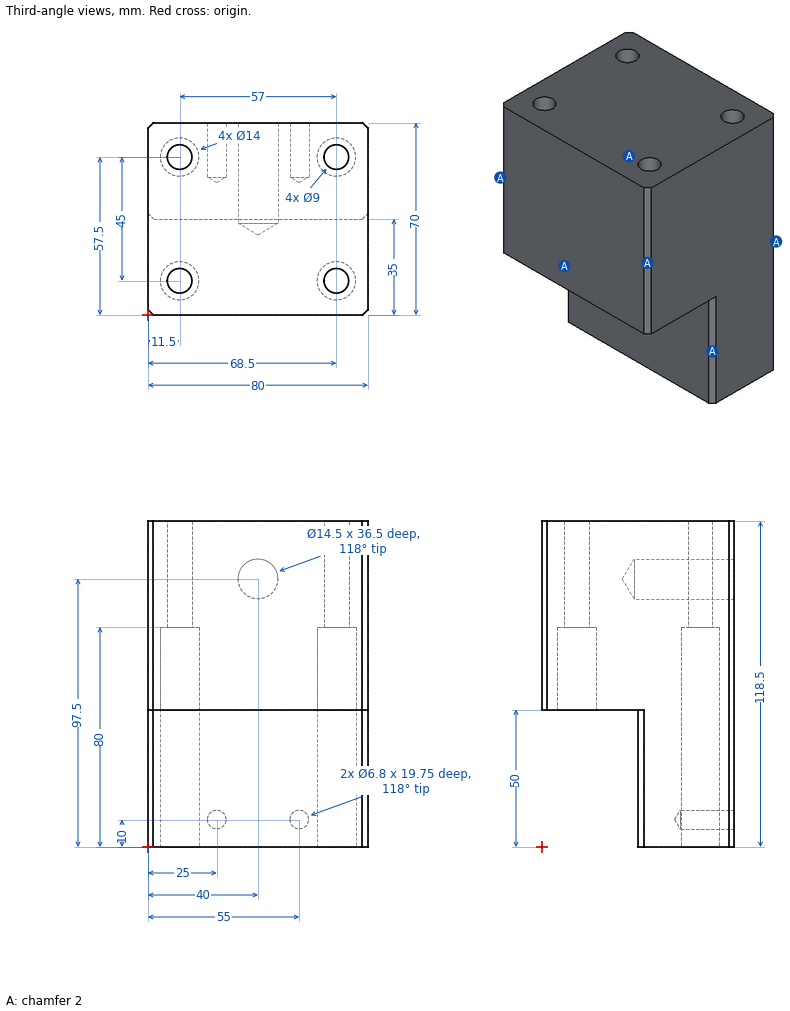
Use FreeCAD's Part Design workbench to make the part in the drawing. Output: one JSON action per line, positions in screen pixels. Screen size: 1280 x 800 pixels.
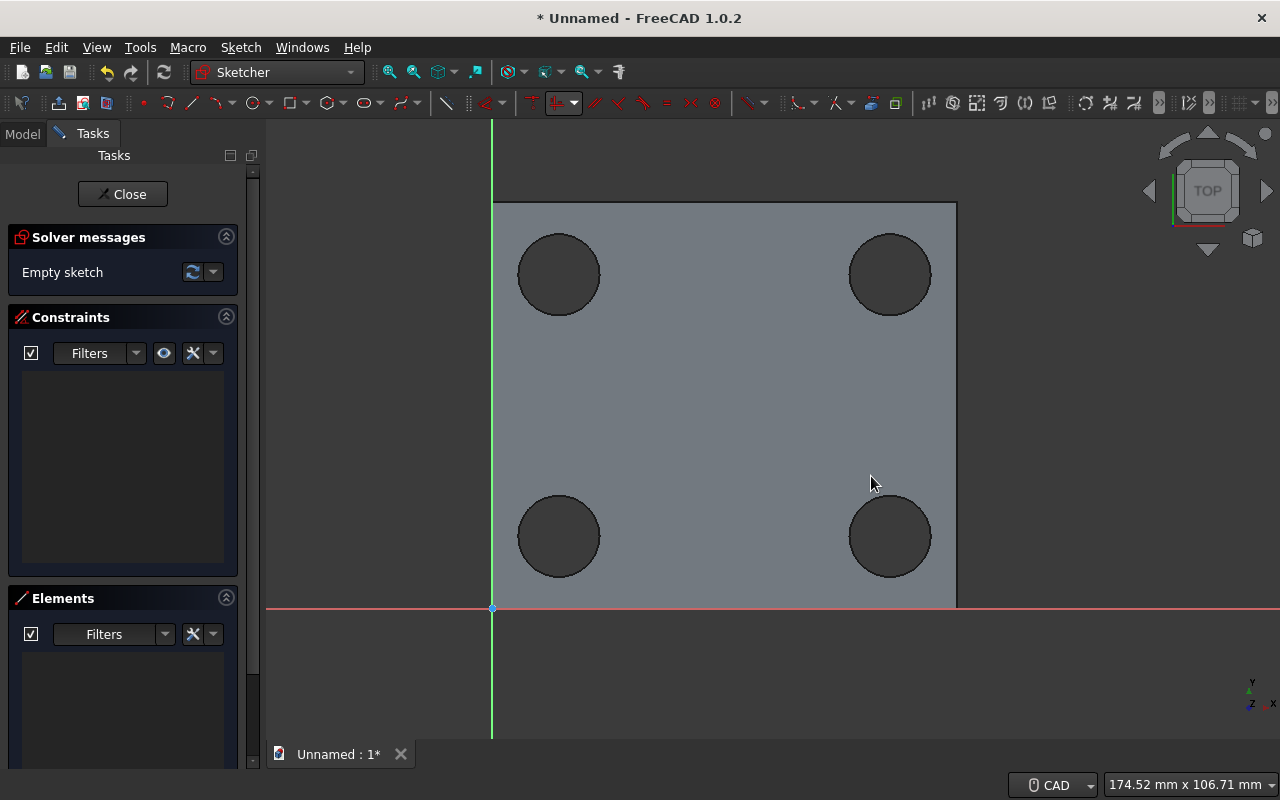
{"action": "left_click", "coordinate": [254, 104]}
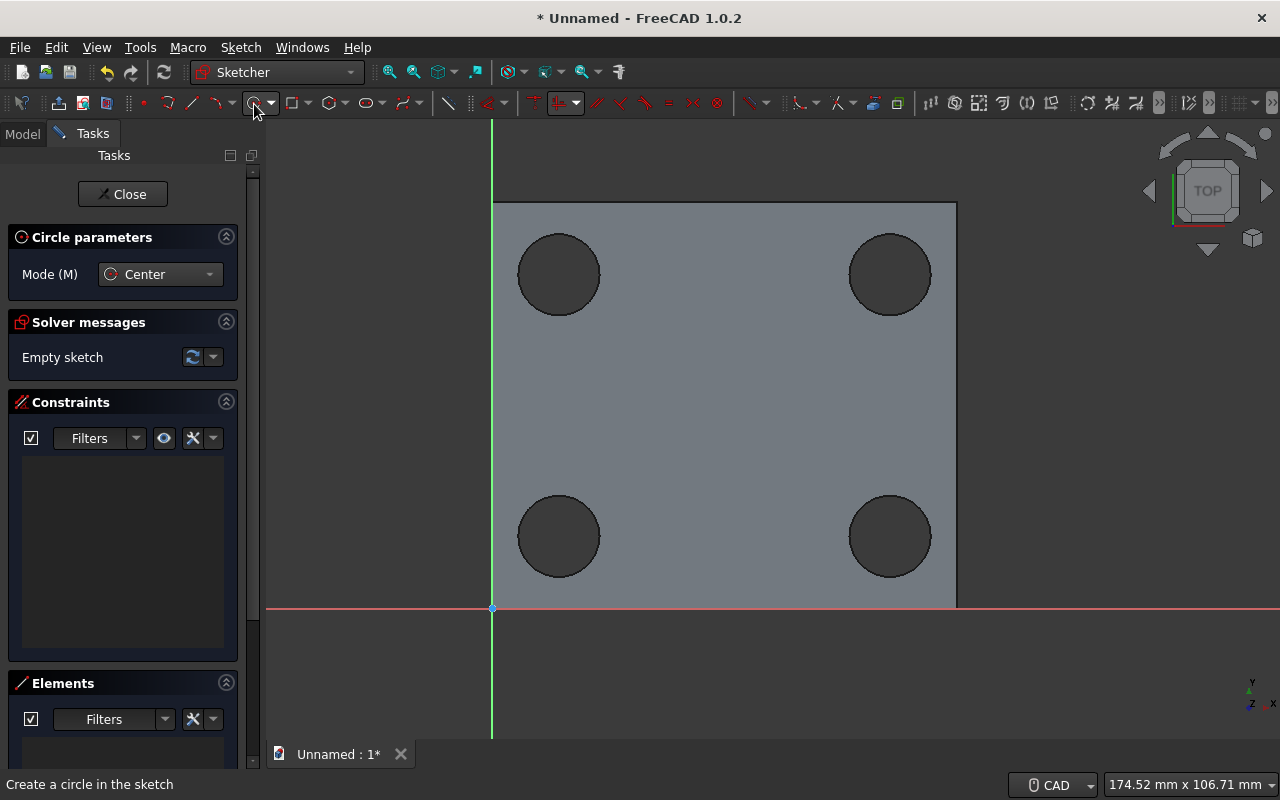
{"action": "left_click", "coordinate": [890, 275]}
{"action": "left_click", "coordinate": [909, 256]}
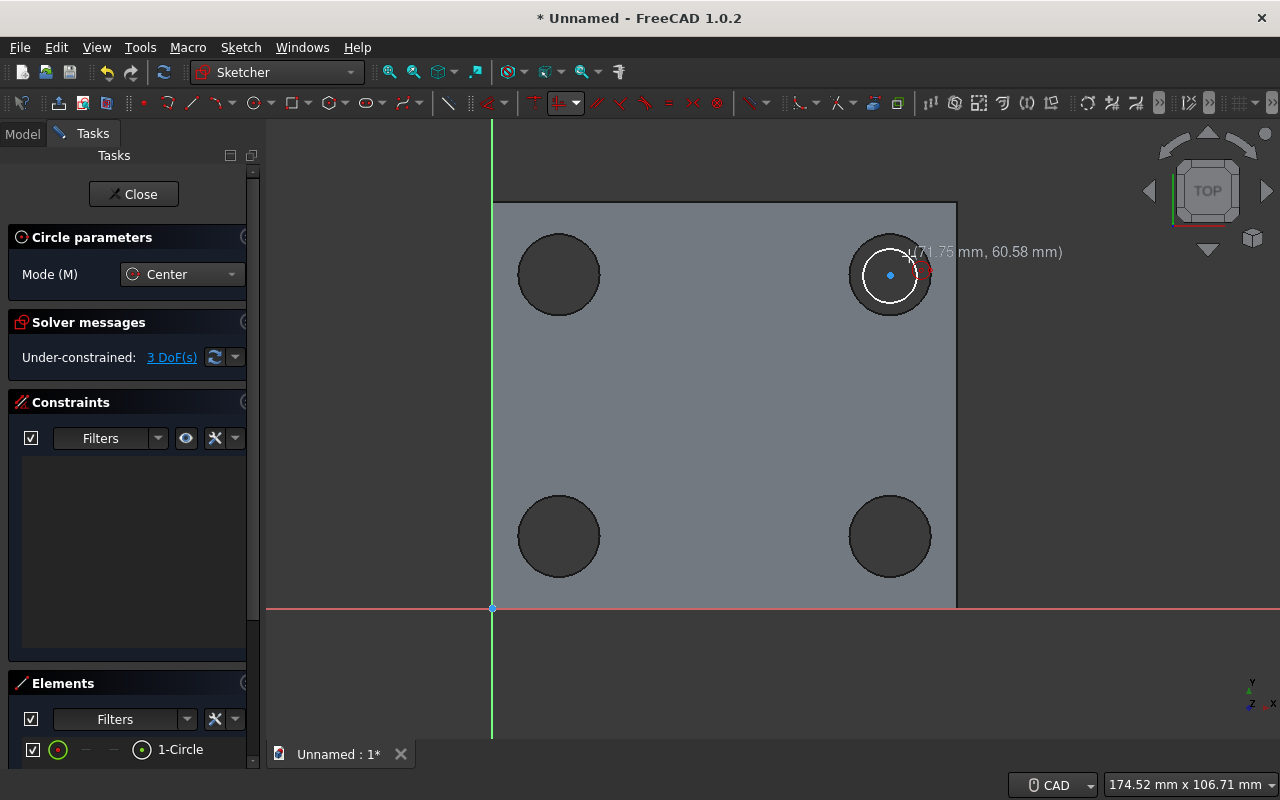
{"action": "left_click", "coordinate": [559, 275]}
{"action": "left_click", "coordinate": [577, 256]}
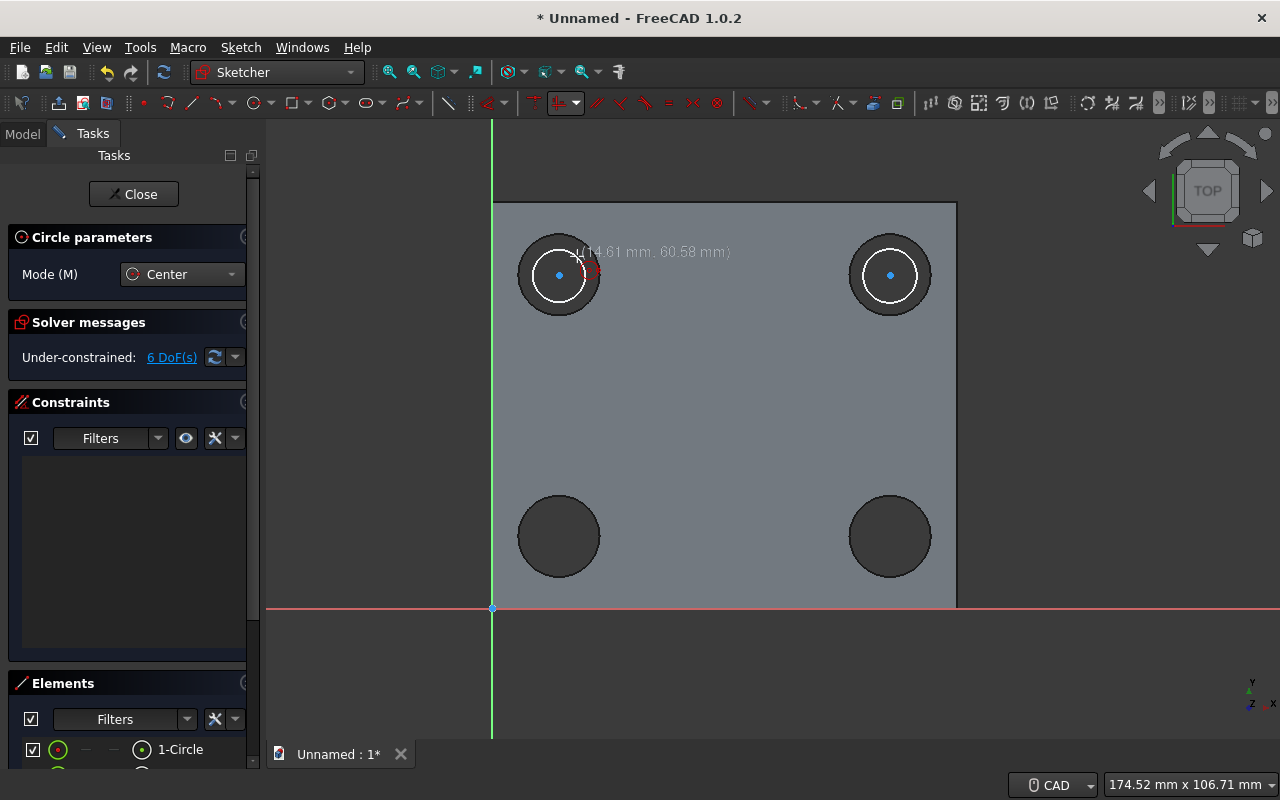
{"action": "left_click", "coordinate": [559, 536]}
{"action": "left_click", "coordinate": [577, 518]}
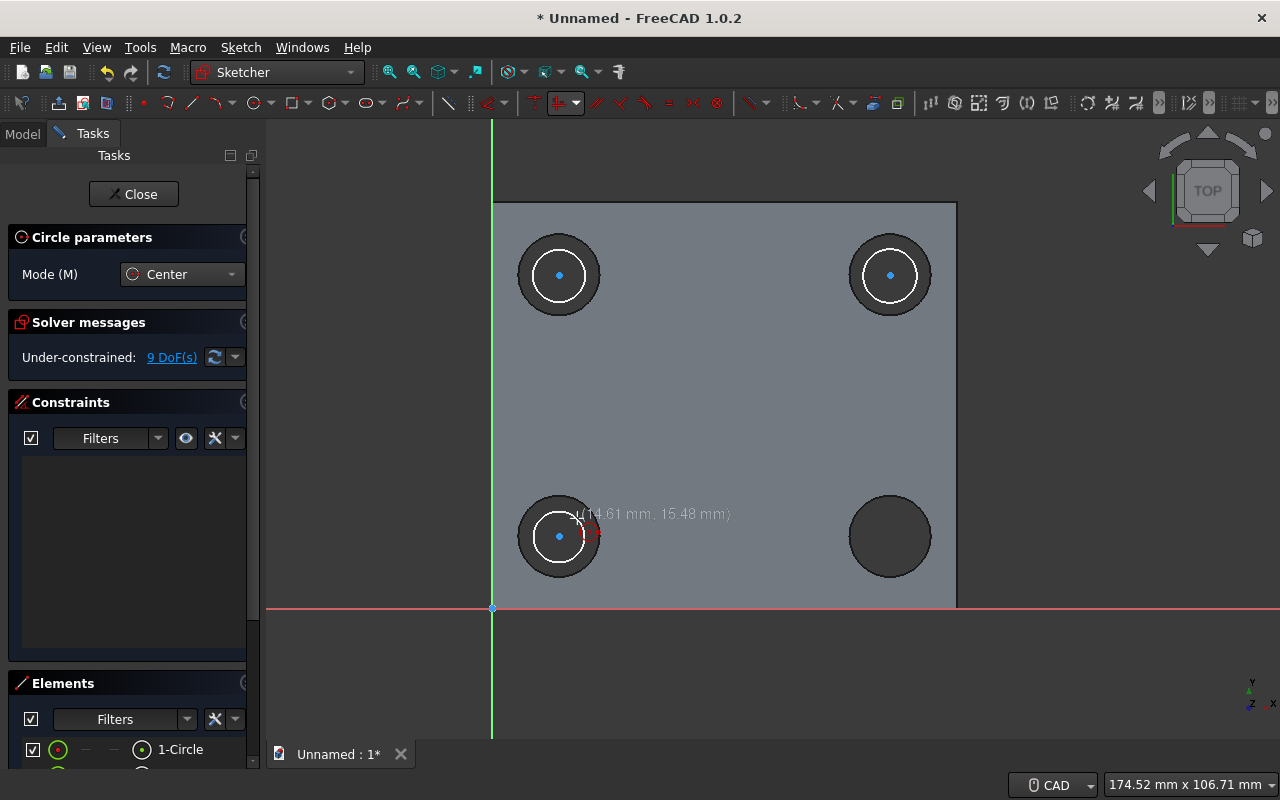
{"action": "left_click", "coordinate": [890, 536]}
{"action": "left_click", "coordinate": [909, 518]}
{"action": "key", "text": "Escape"}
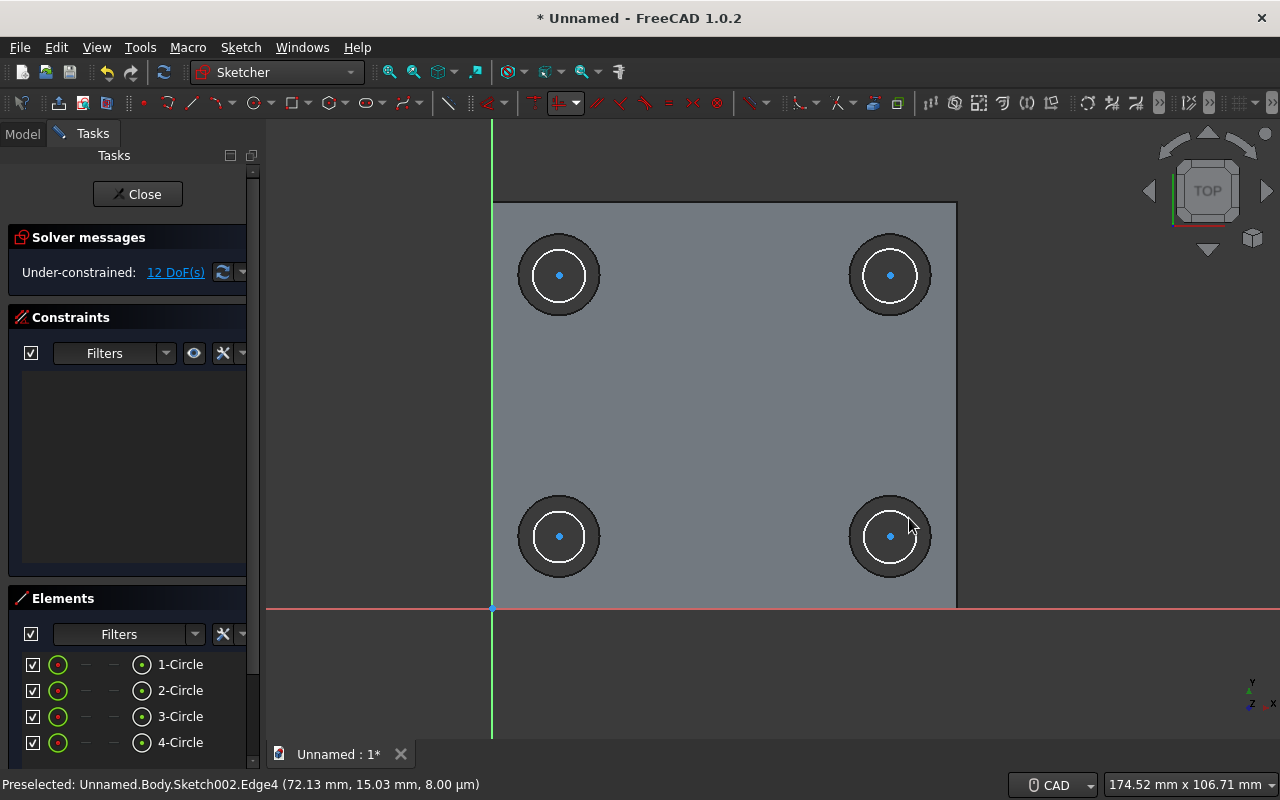
{"action": "left_click", "coordinate": [909, 257]}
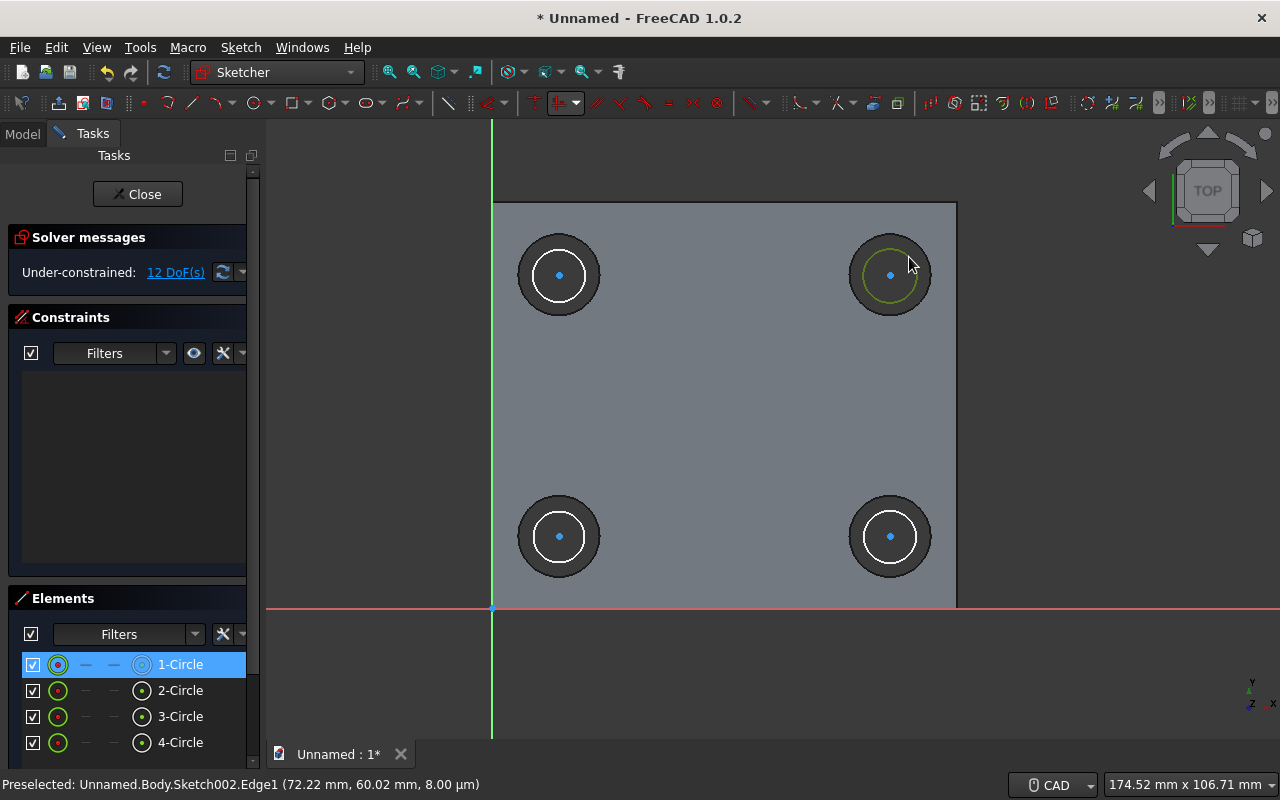
{"action": "left_click", "coordinate": [577, 257]}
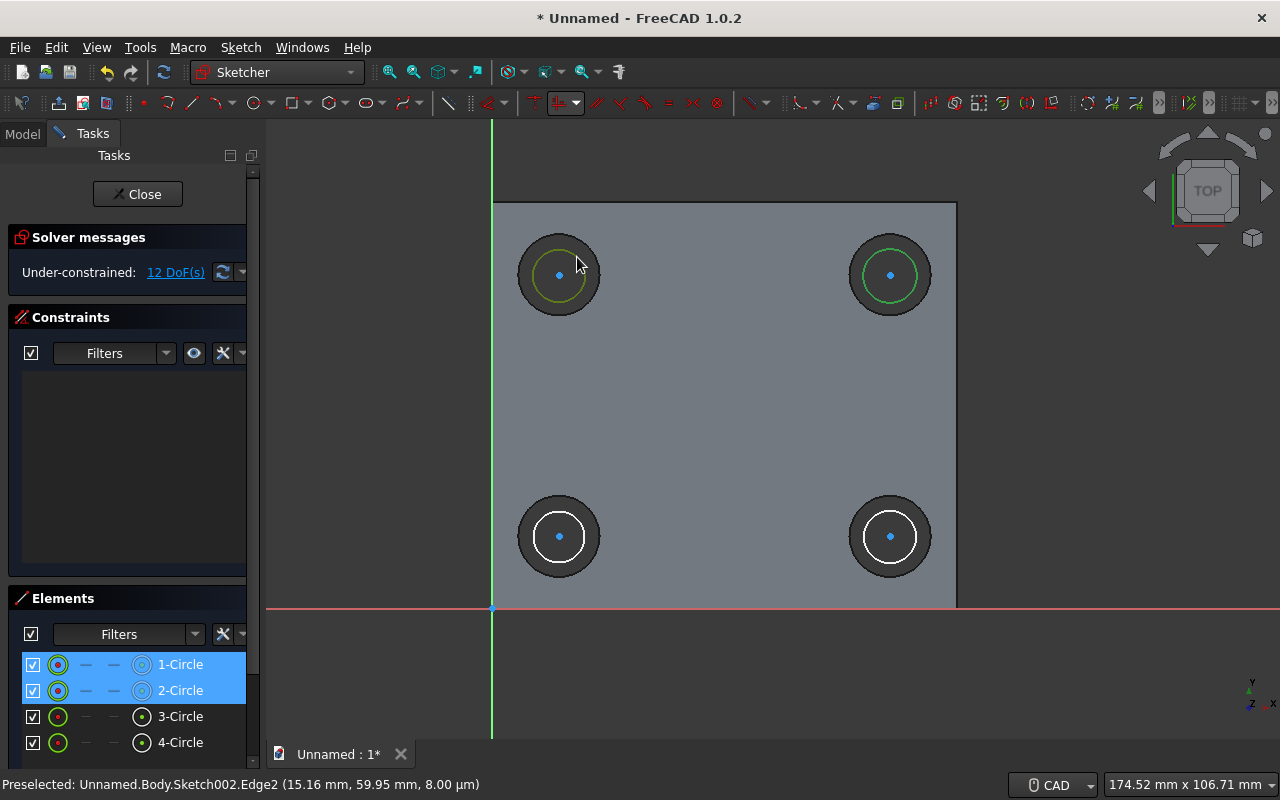
{"action": "left_click", "coordinate": [577, 519]}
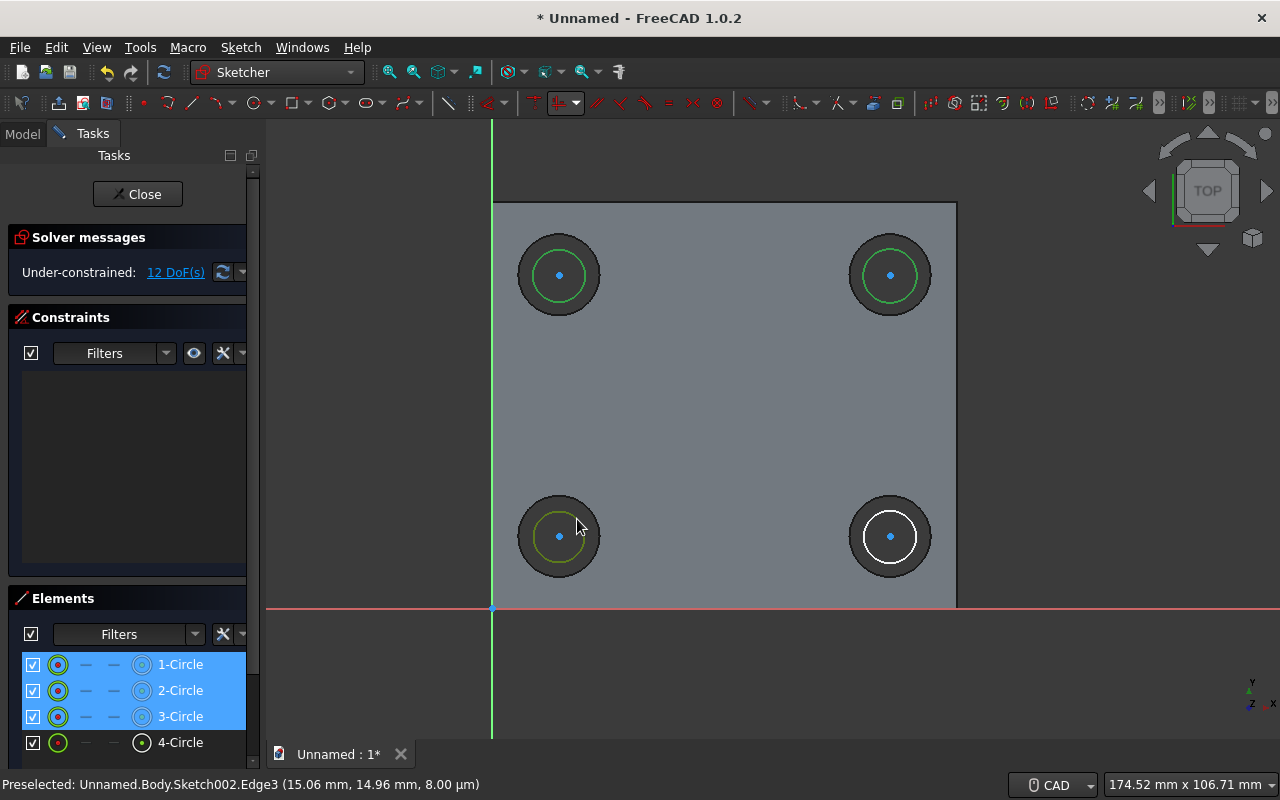
{"action": "left_click", "coordinate": [908, 518]}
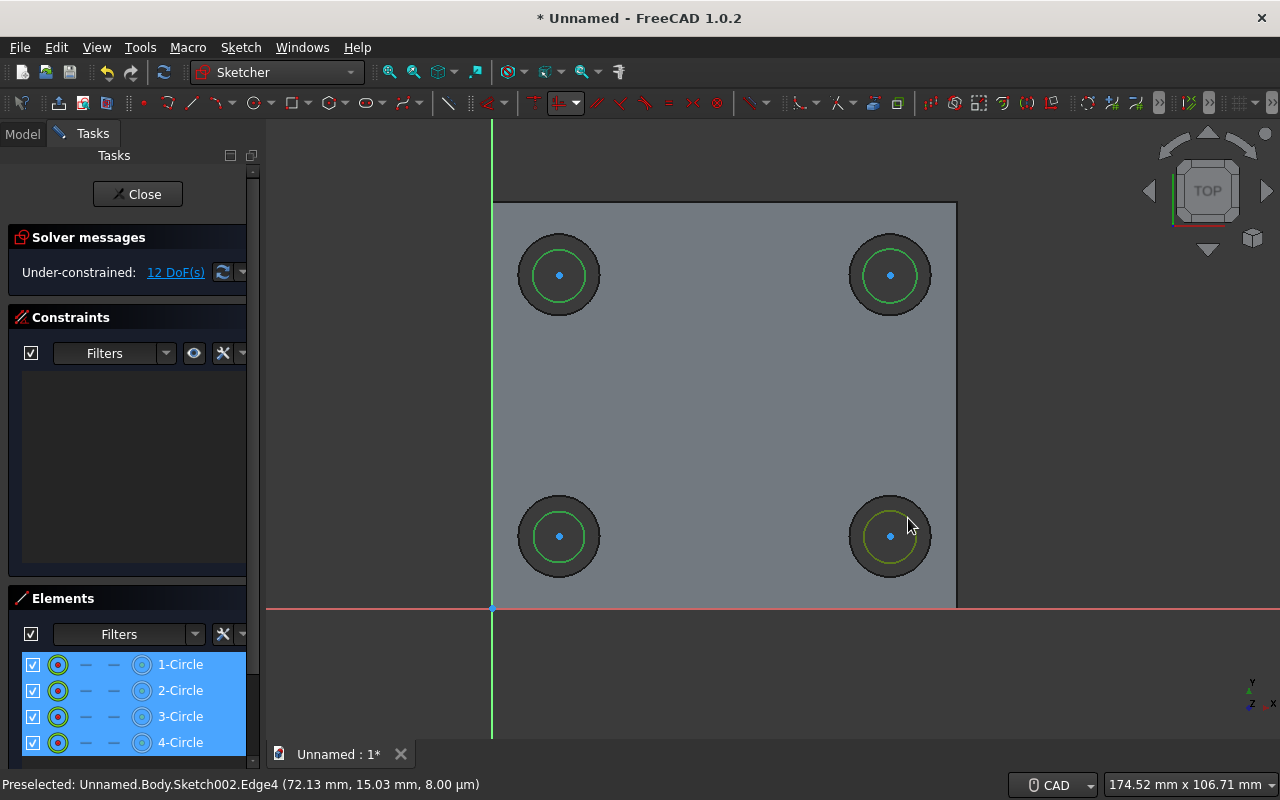
{"action": "key", "text": "e"}